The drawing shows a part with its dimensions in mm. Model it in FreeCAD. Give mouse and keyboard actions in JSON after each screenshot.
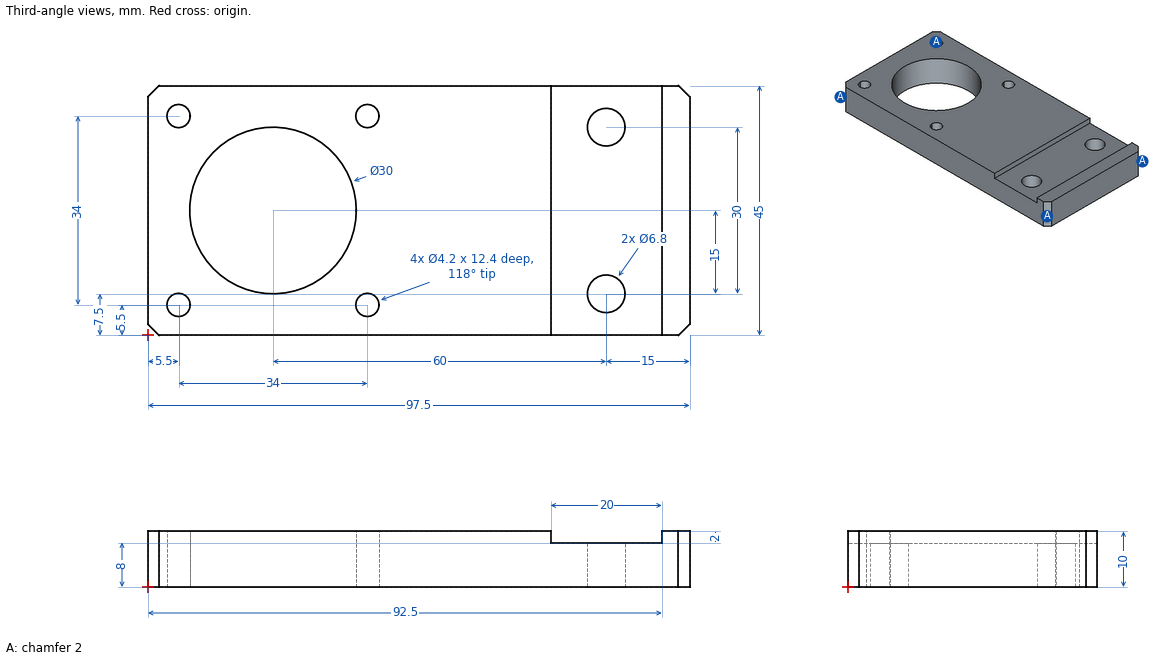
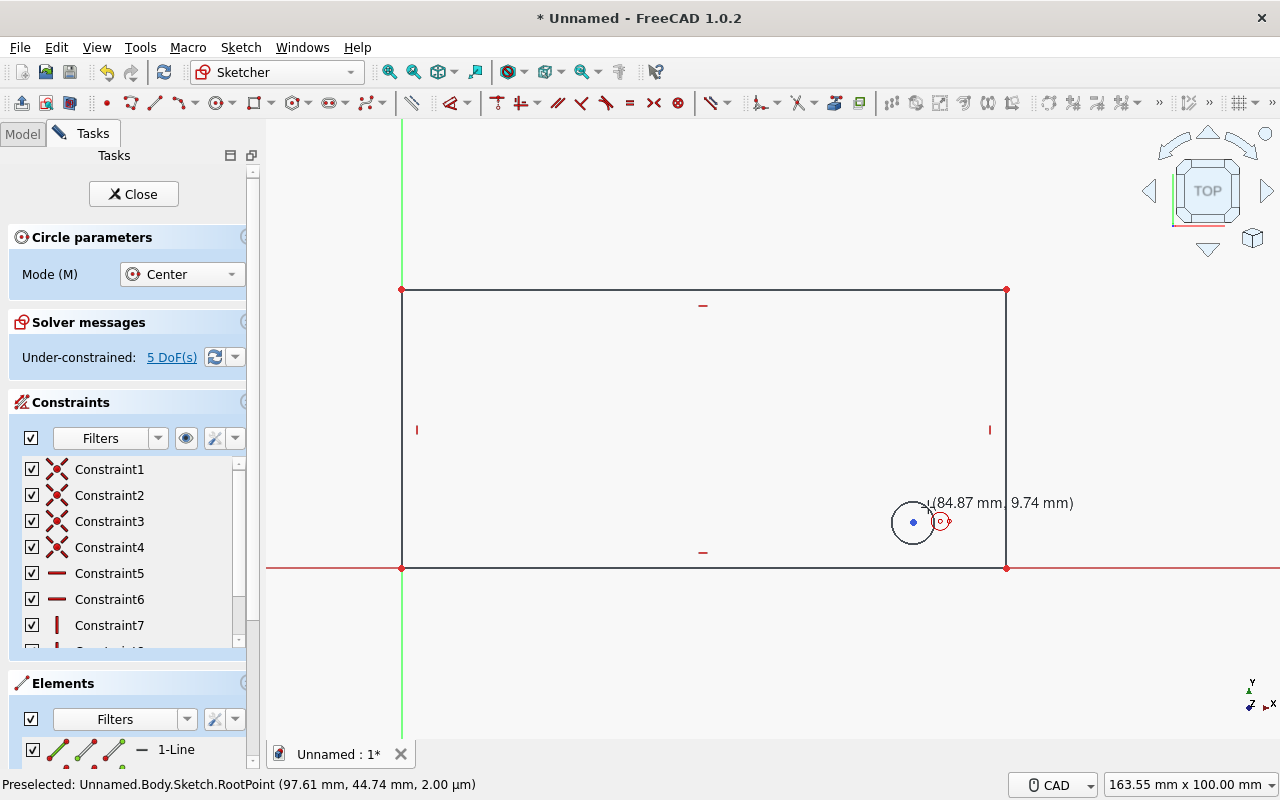
{"action": "left_click", "coordinate": [541, 429]}
{"action": "left_click", "coordinate": [607, 363]}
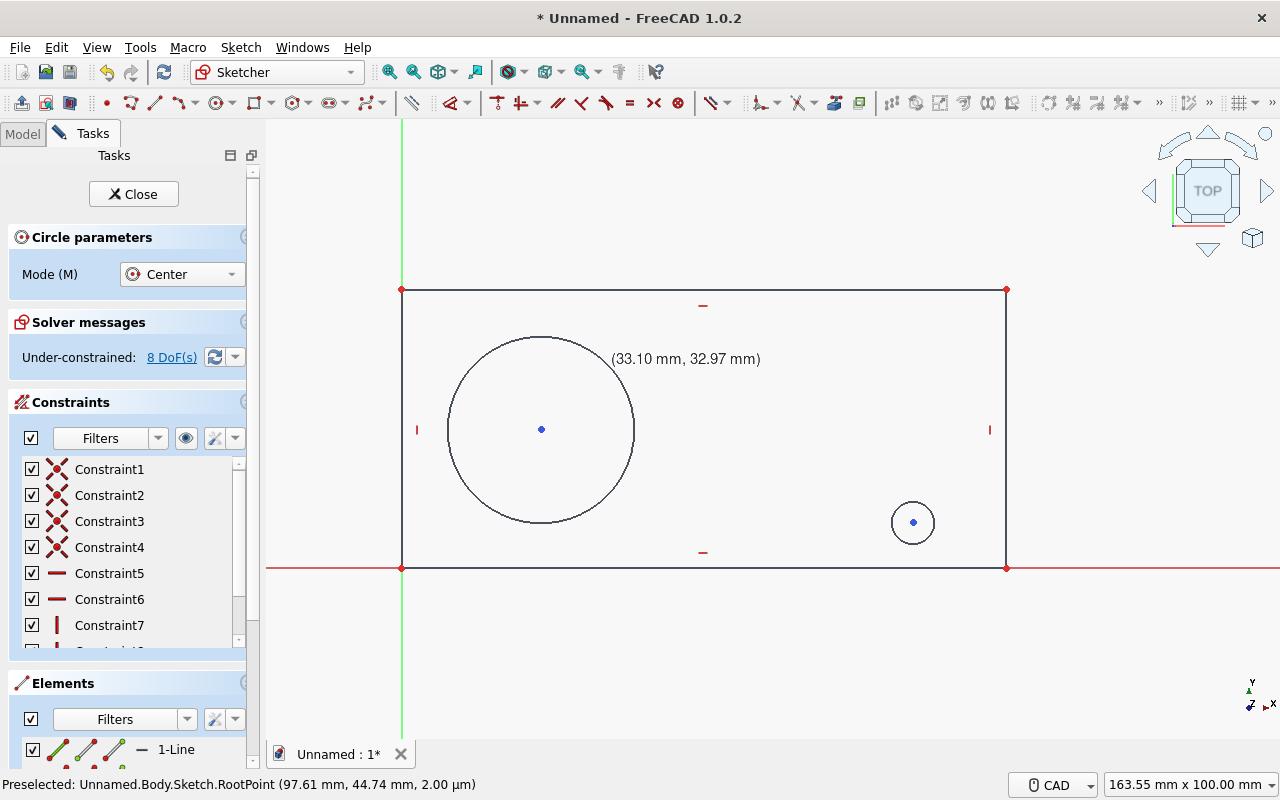
{"action": "left_click", "coordinate": [913, 336]}
{"action": "left_click", "coordinate": [928, 321]}
{"action": "key", "text": "Escape"}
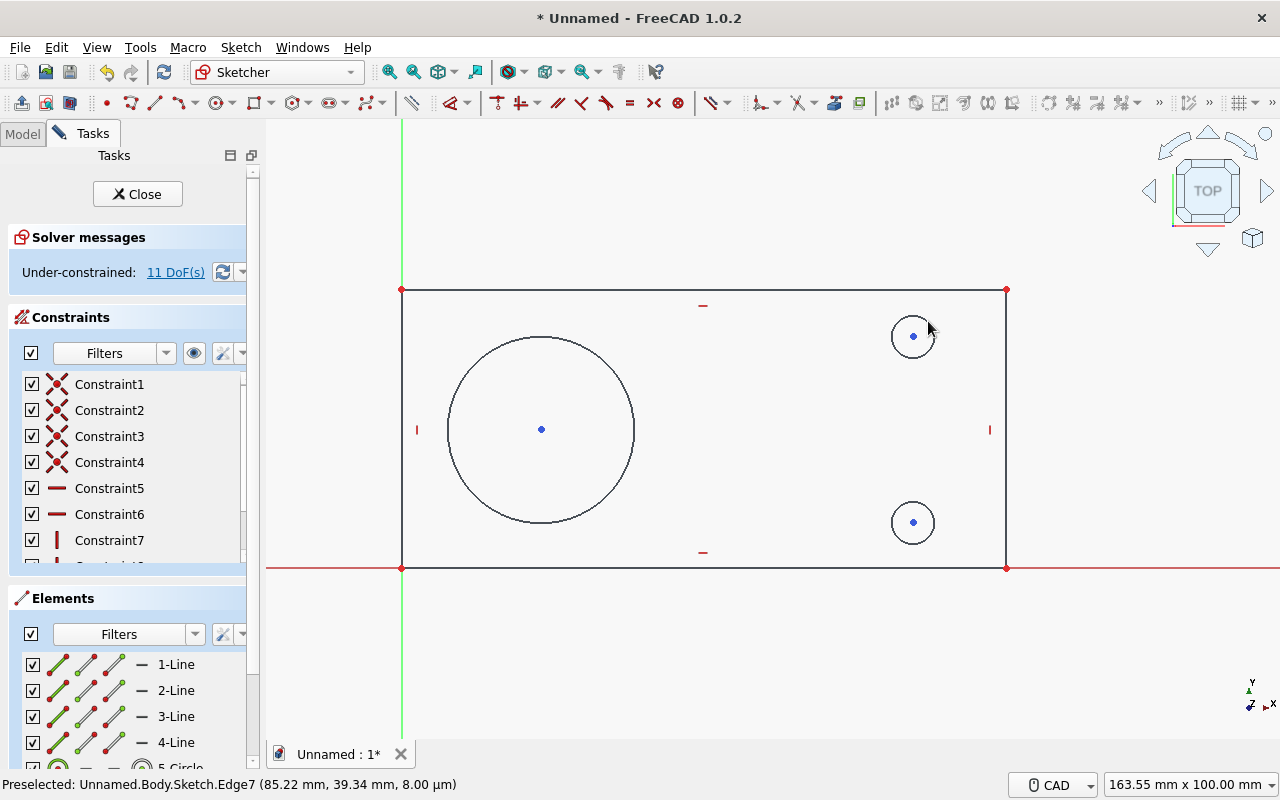
{"action": "left_click", "coordinate": [928, 508]}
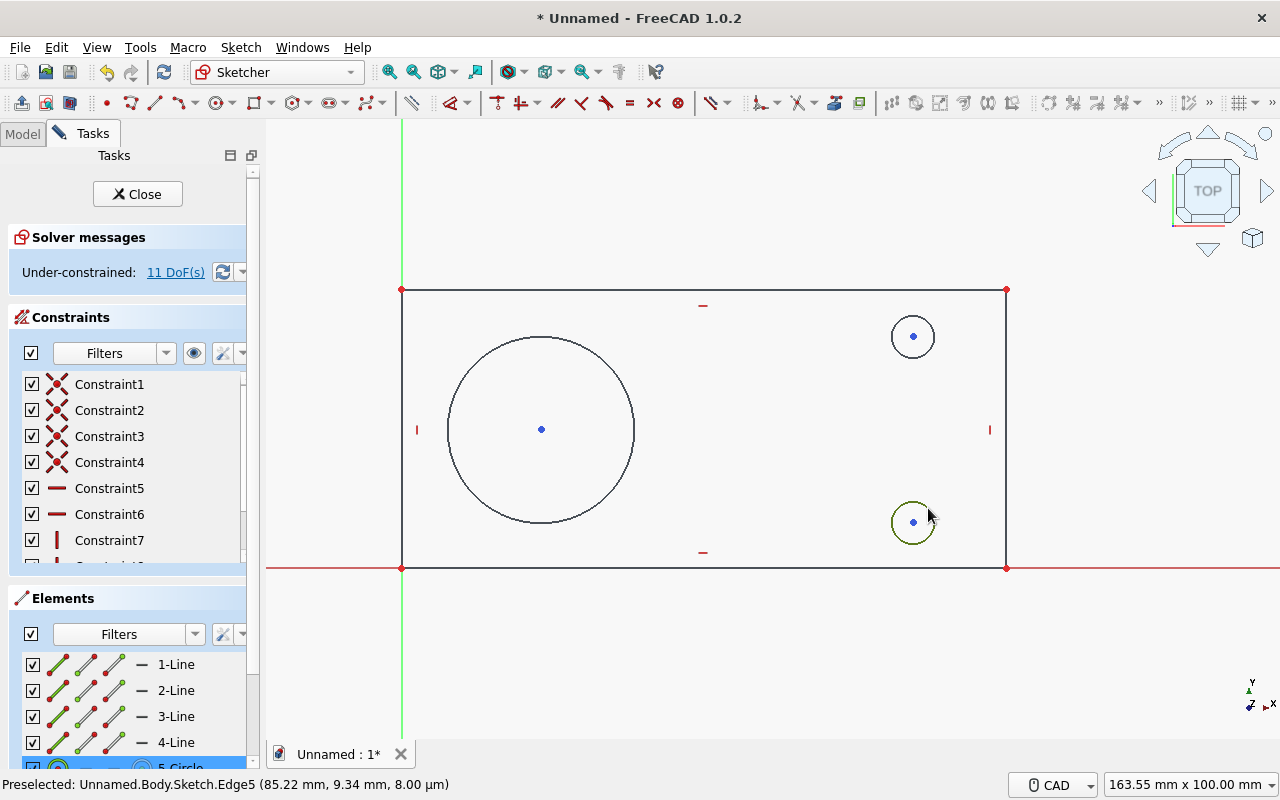
{"action": "left_click", "coordinate": [928, 322]}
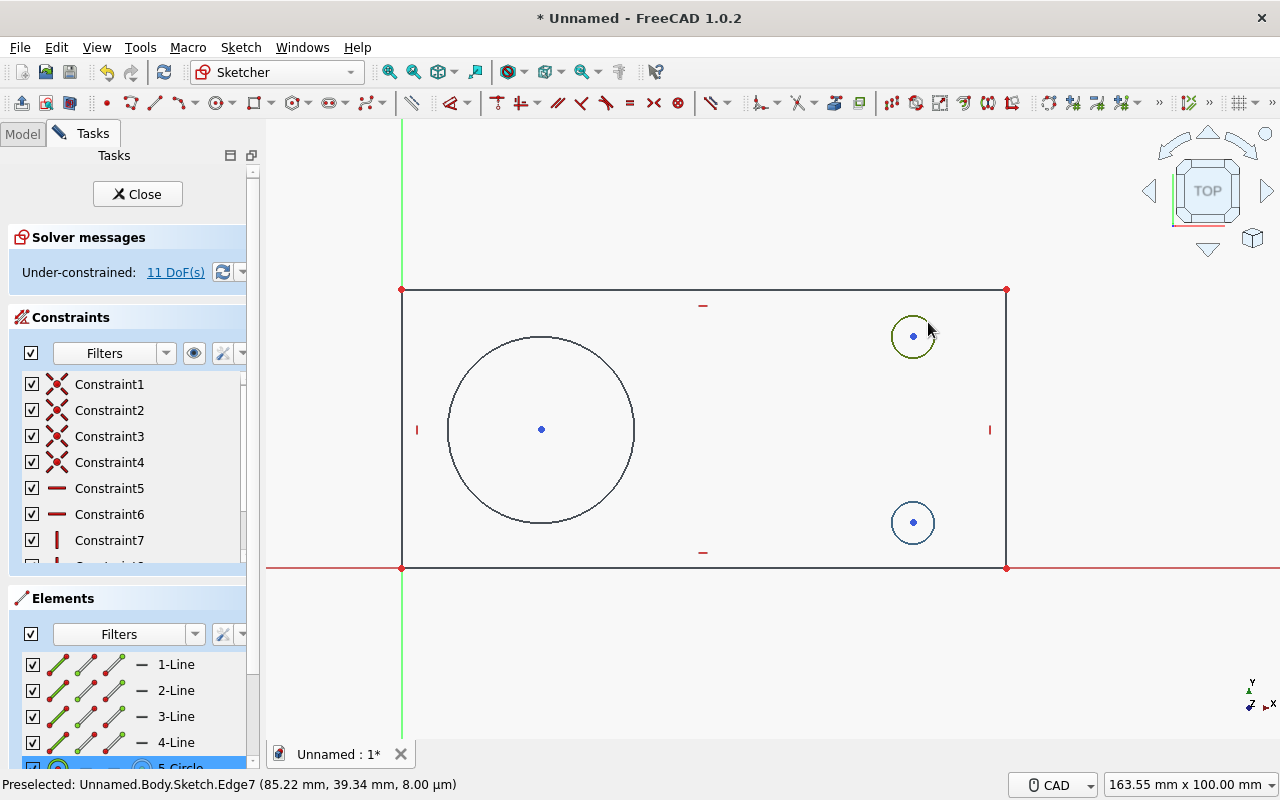
{"action": "left_click", "coordinate": [630, 104]}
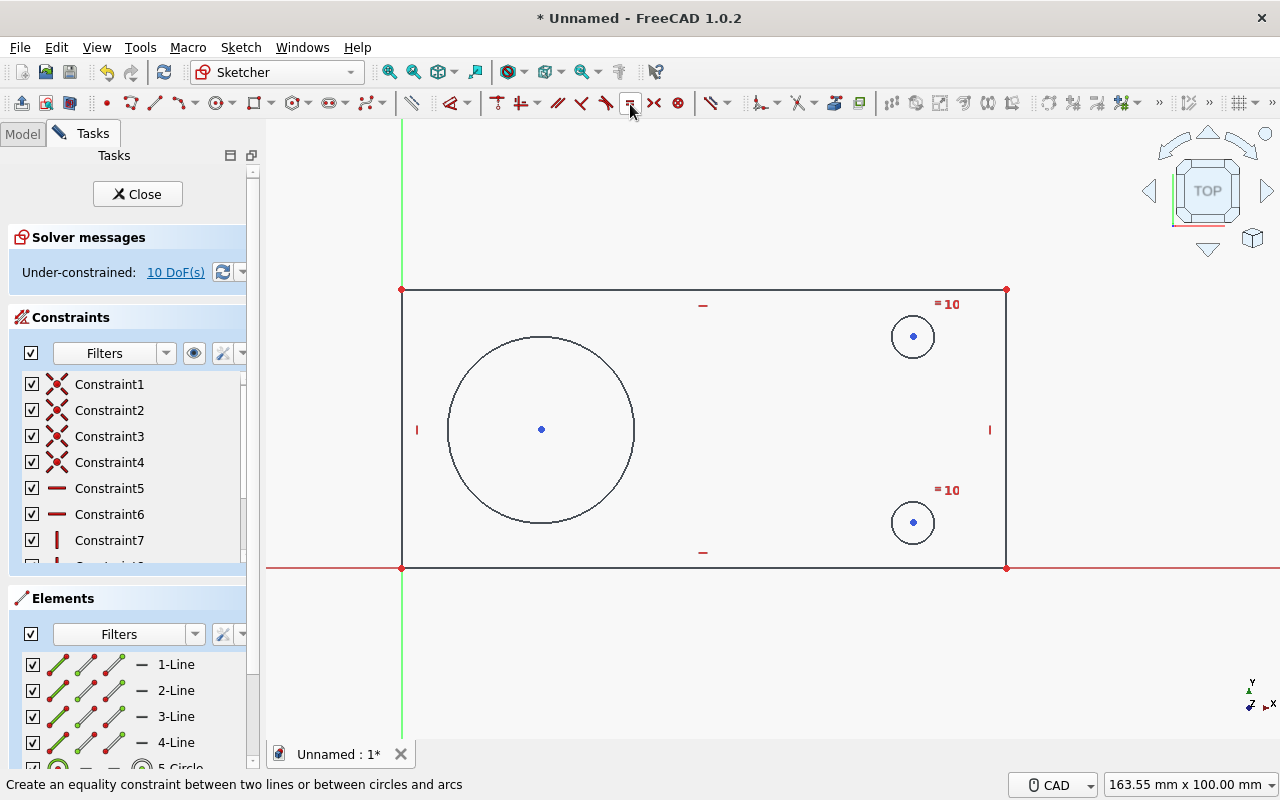
{"action": "left_click", "coordinate": [913, 523]}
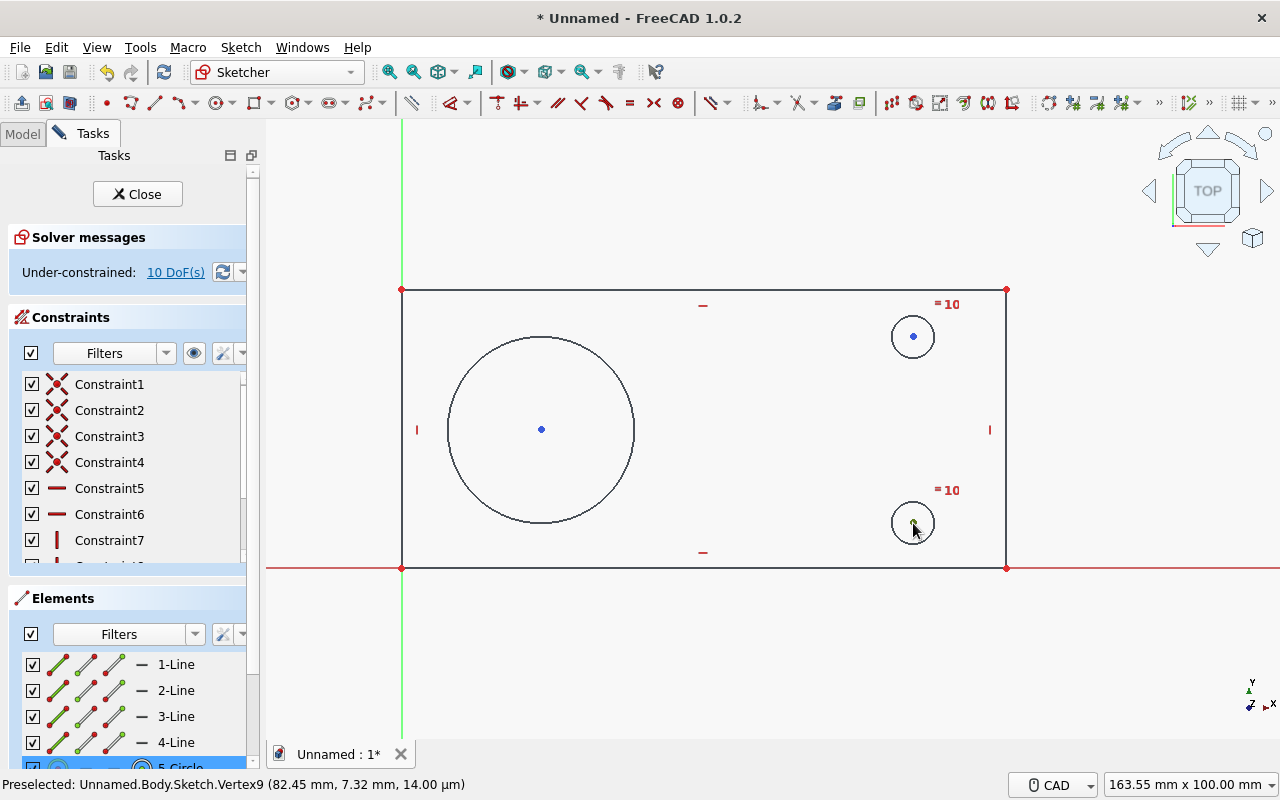
{"action": "left_click", "coordinate": [913, 337]}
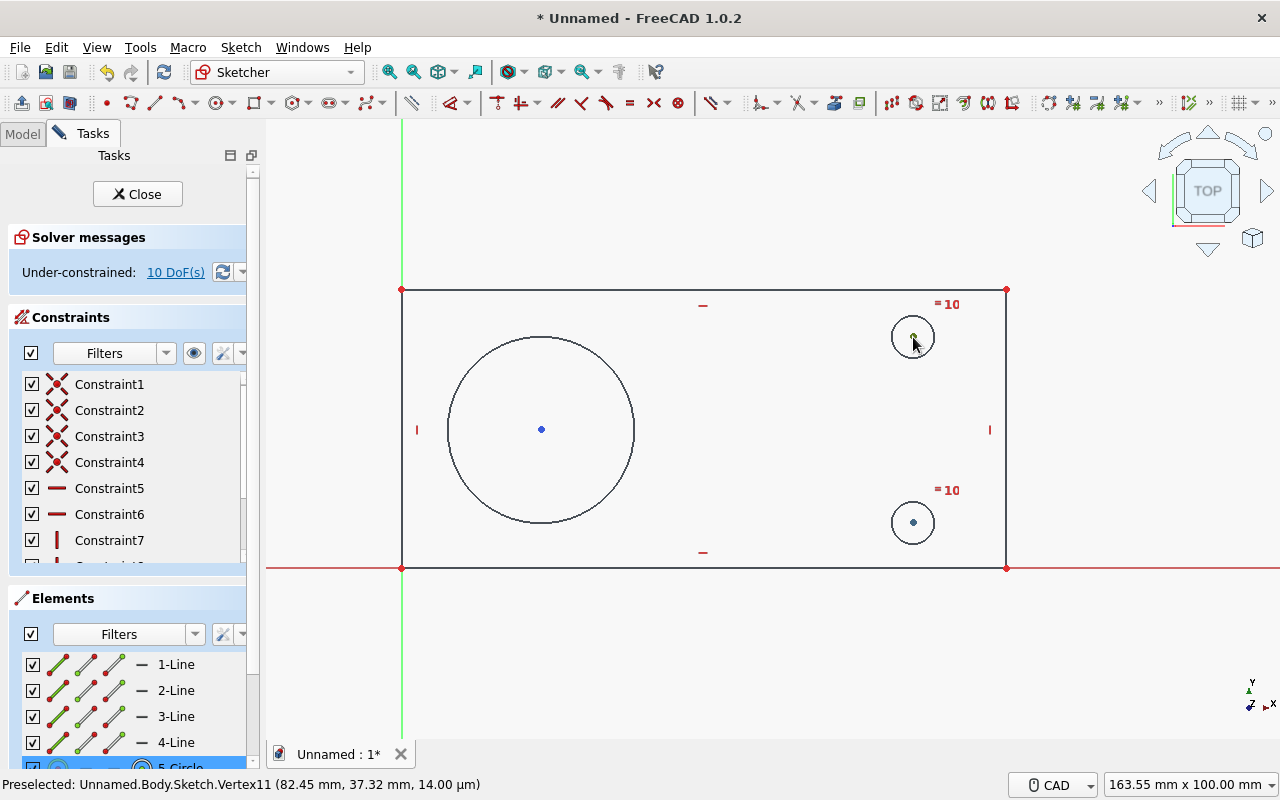
{"action": "key", "text": "v"}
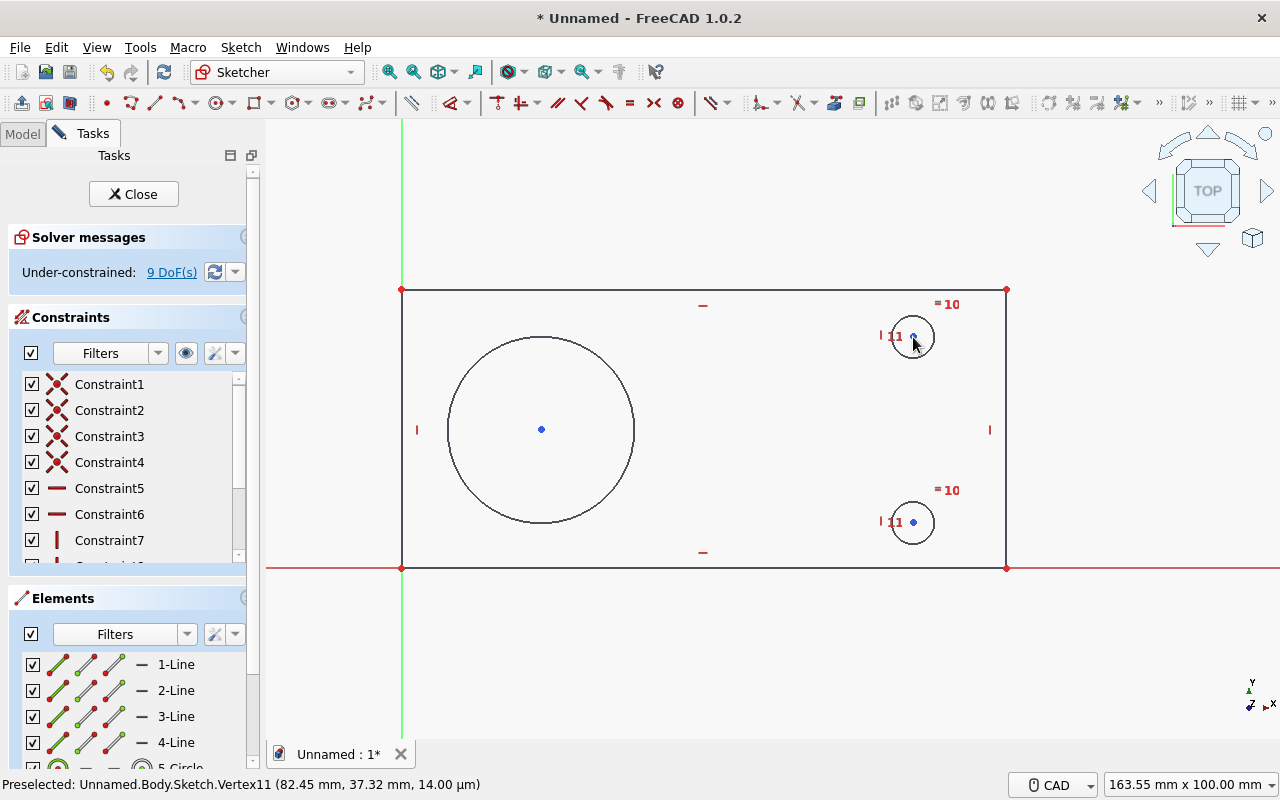
{"action": "left_click", "coordinate": [928, 508]}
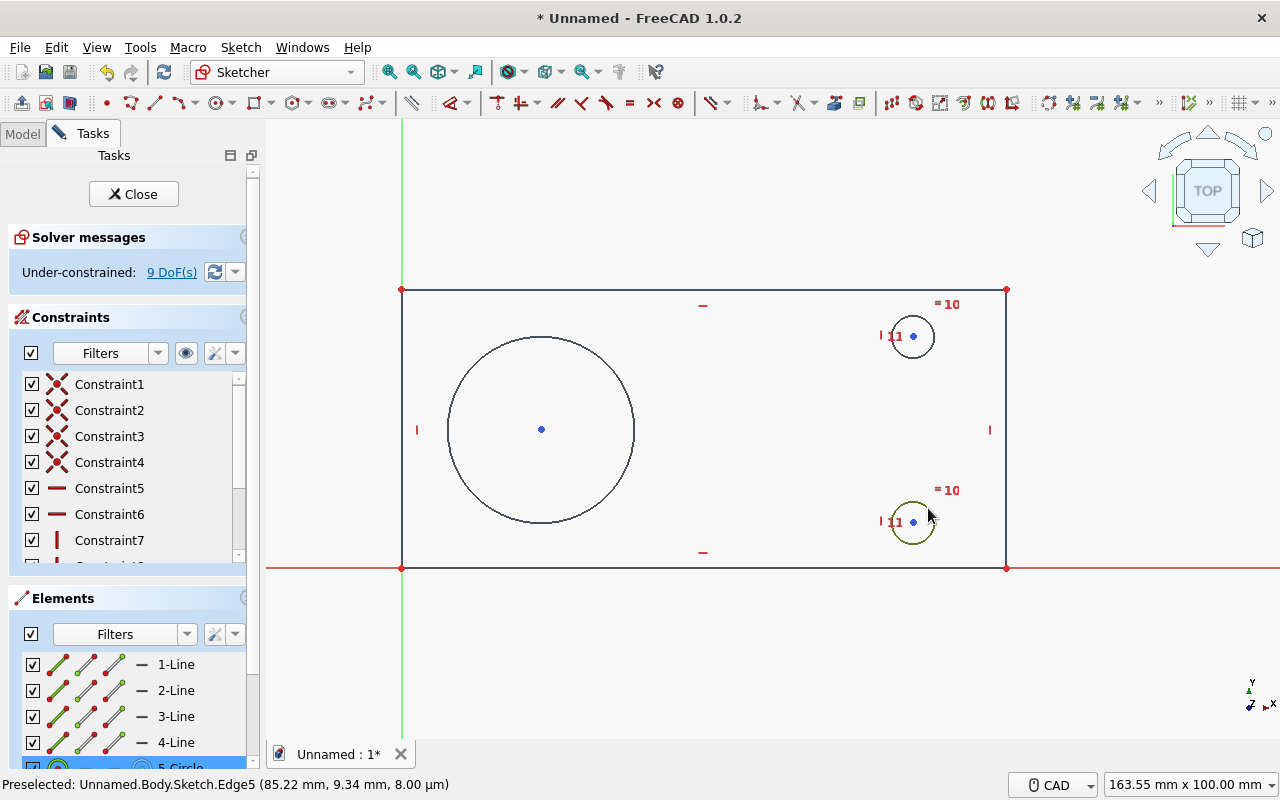
{"action": "left_click", "coordinate": [470, 104]}